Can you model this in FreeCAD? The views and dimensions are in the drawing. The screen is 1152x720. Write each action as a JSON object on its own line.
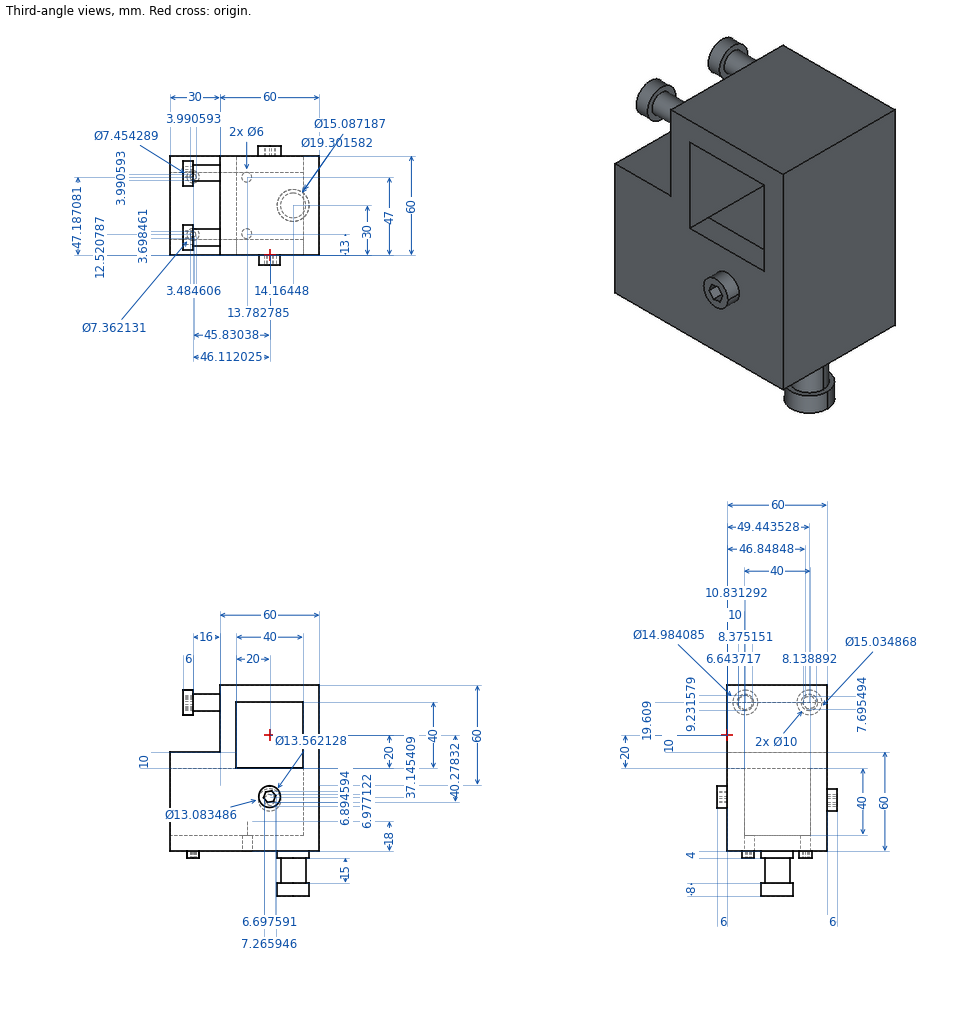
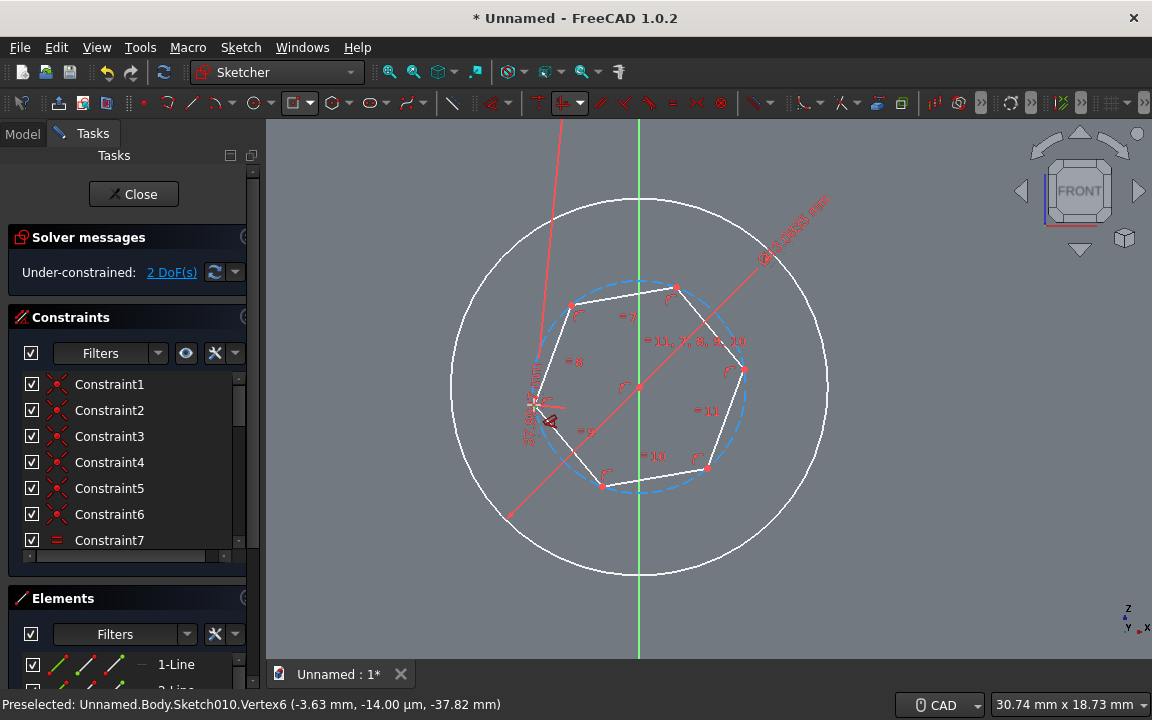
{"action": "left_click", "coordinate": [744, 369]}
{"action": "left_click", "coordinate": [591, 439]}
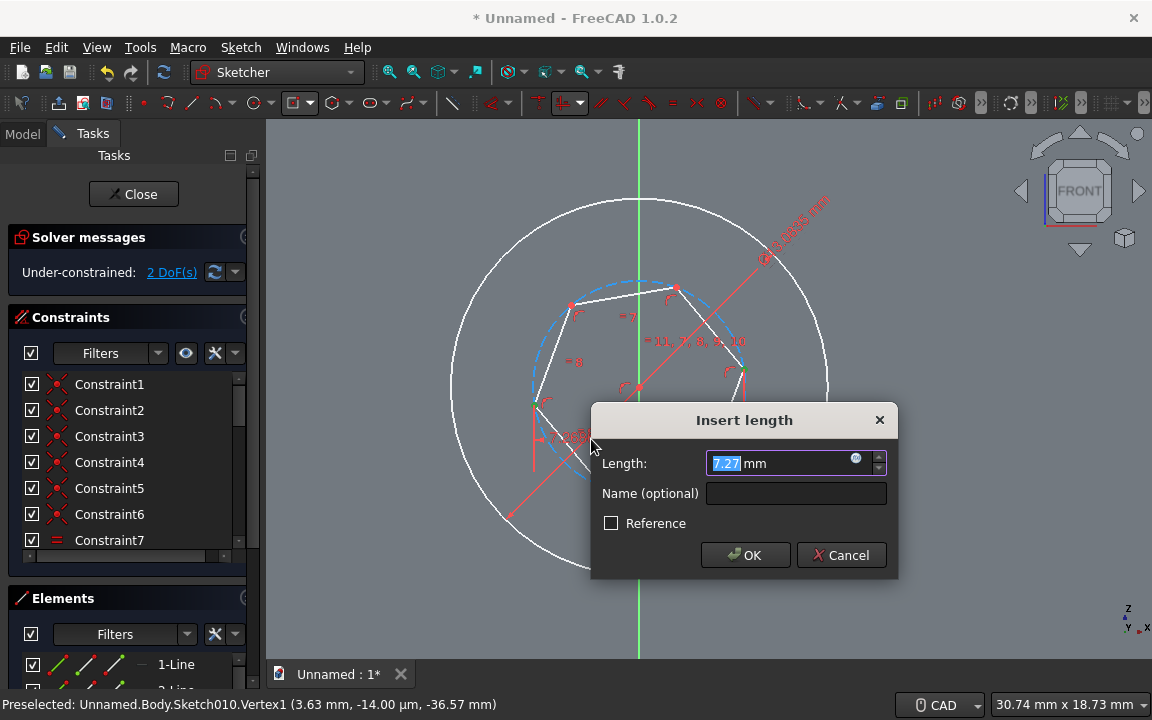
{"action": "type", "text": "7.265946"}
{"action": "key", "text": "Return"}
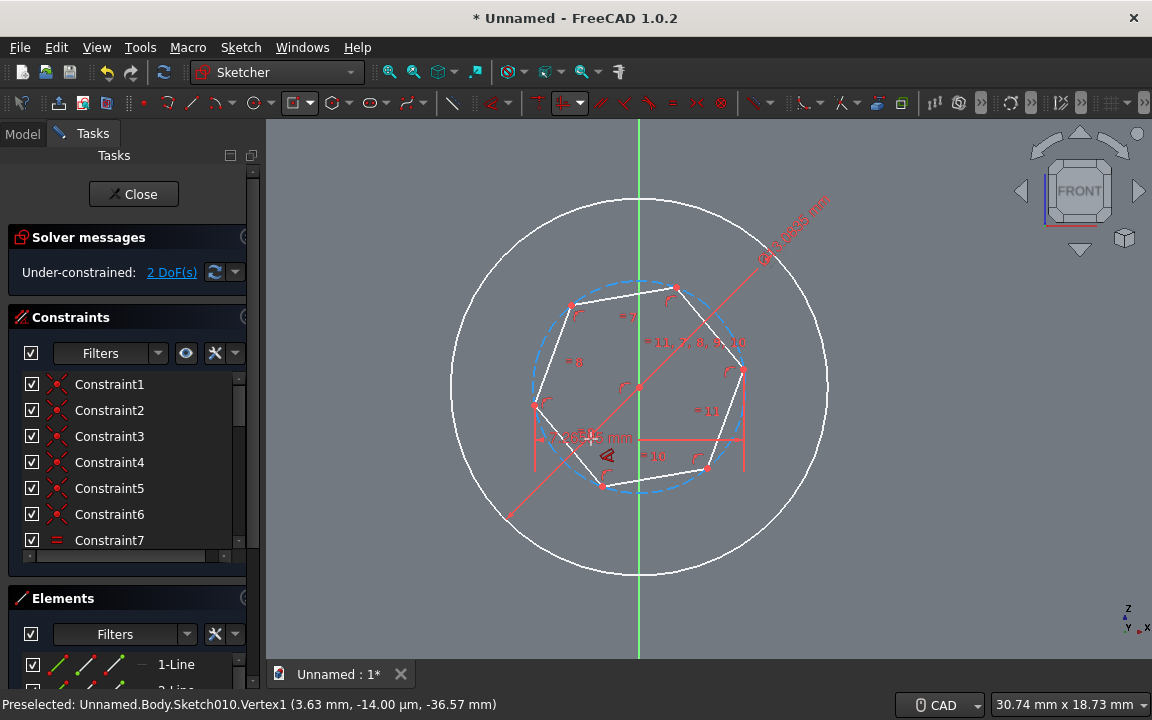
{"action": "left_click", "coordinate": [602, 487]}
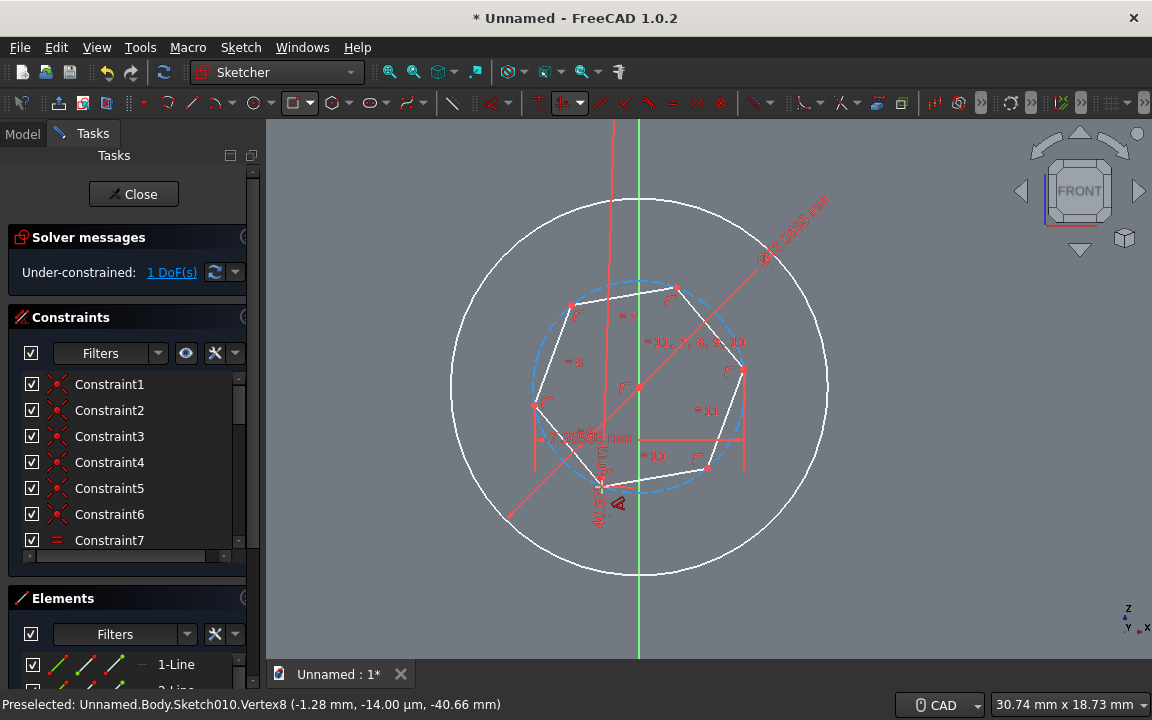
{"action": "left_click", "coordinate": [676, 287]}
{"action": "left_click", "coordinate": [710, 387]}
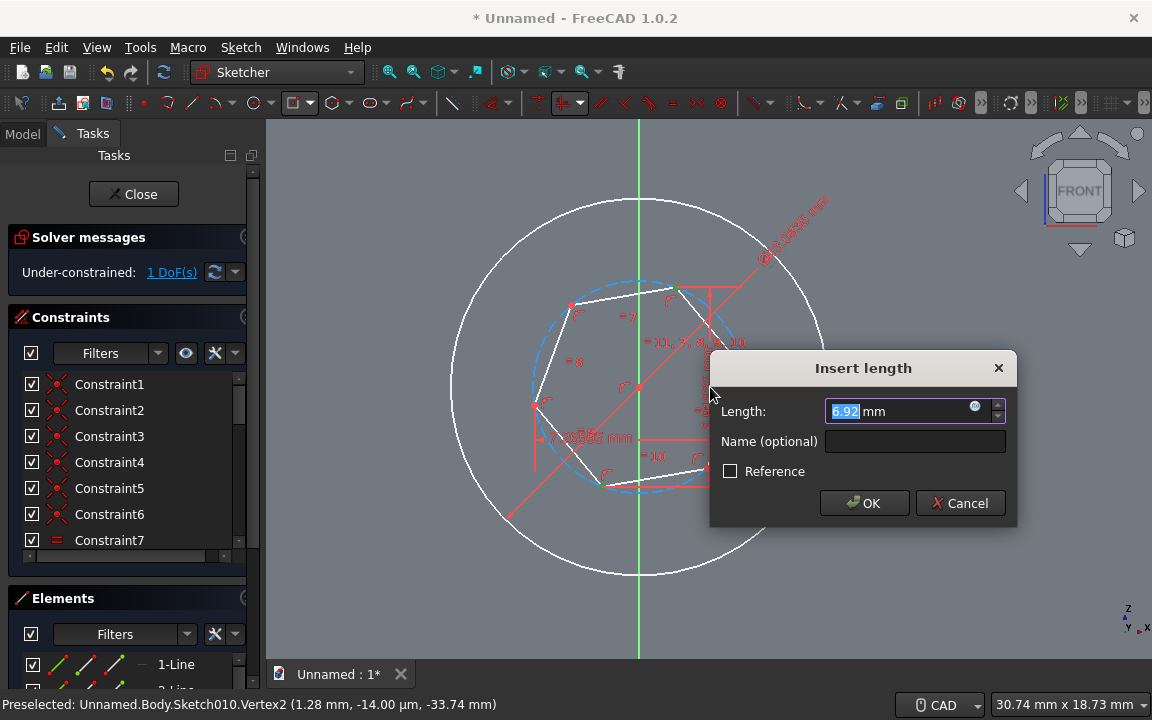
{"action": "type", "text": "6.894594"}
{"action": "key", "text": "Return"}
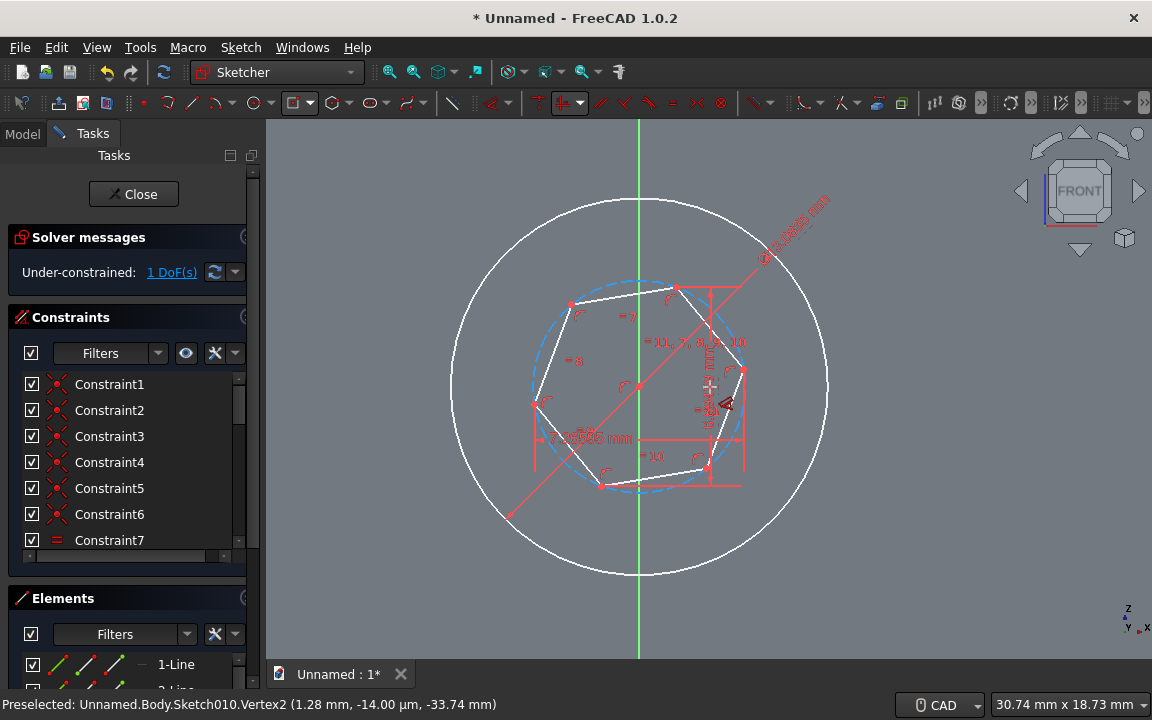
{"action": "left_click", "coordinate": [639, 387]}
{"action": "left_click", "coordinate": [673, 267]}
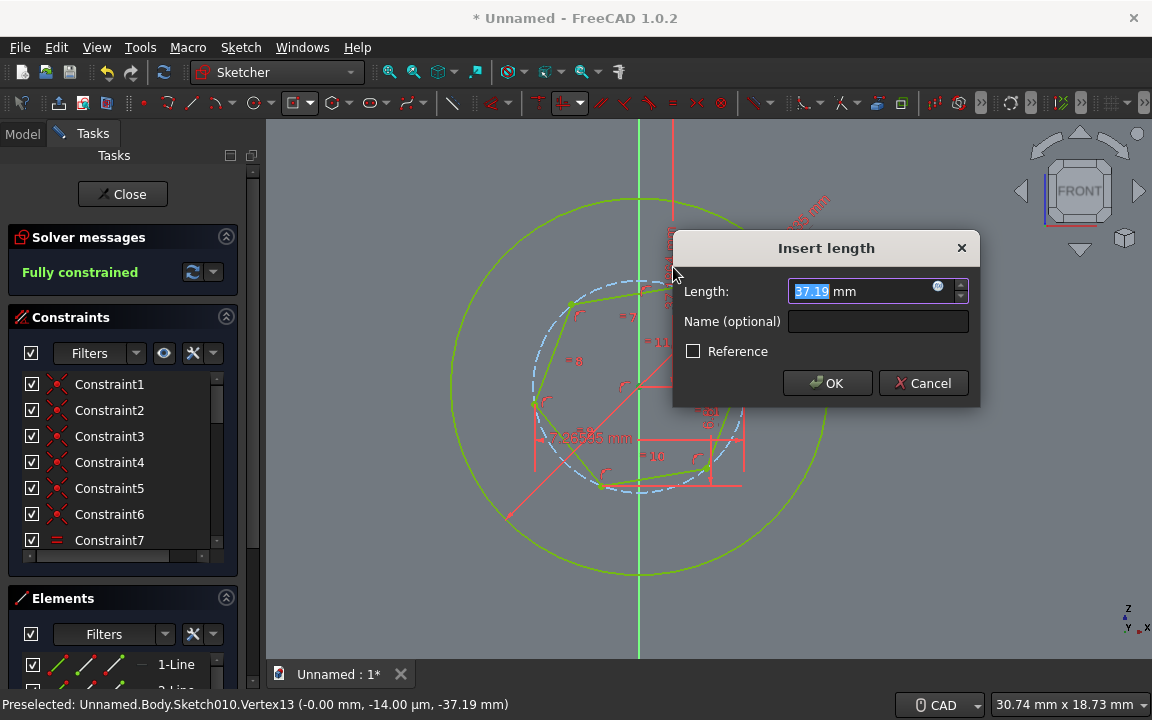
{"action": "type", "text": "37.145409"}
{"action": "key", "text": "Return"}
{"action": "key", "text": "Escape"}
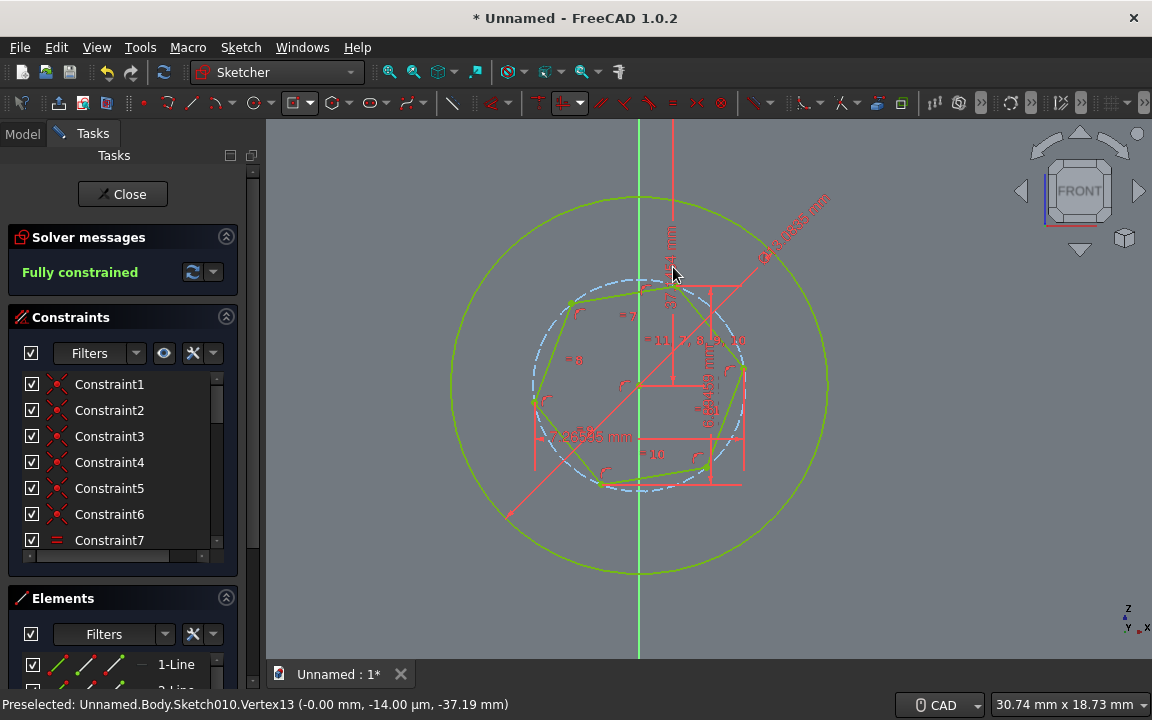
{"action": "left_click", "coordinate": [123, 194]}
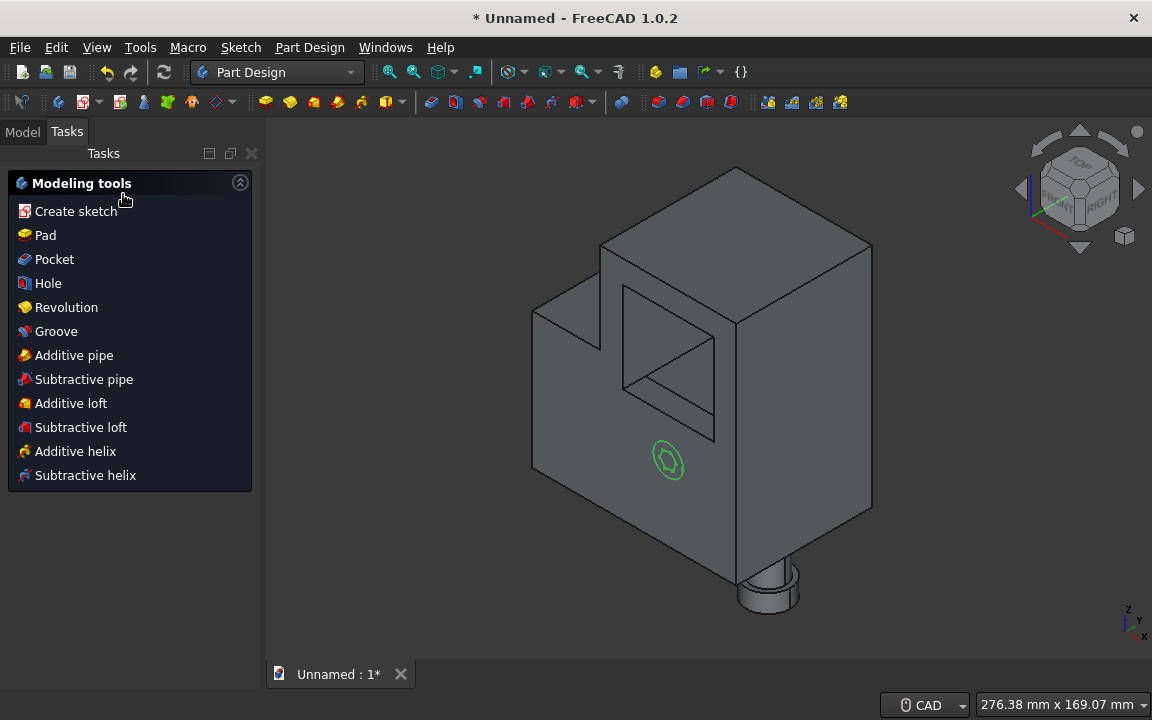
{"action": "left_click", "coordinate": [266, 102]}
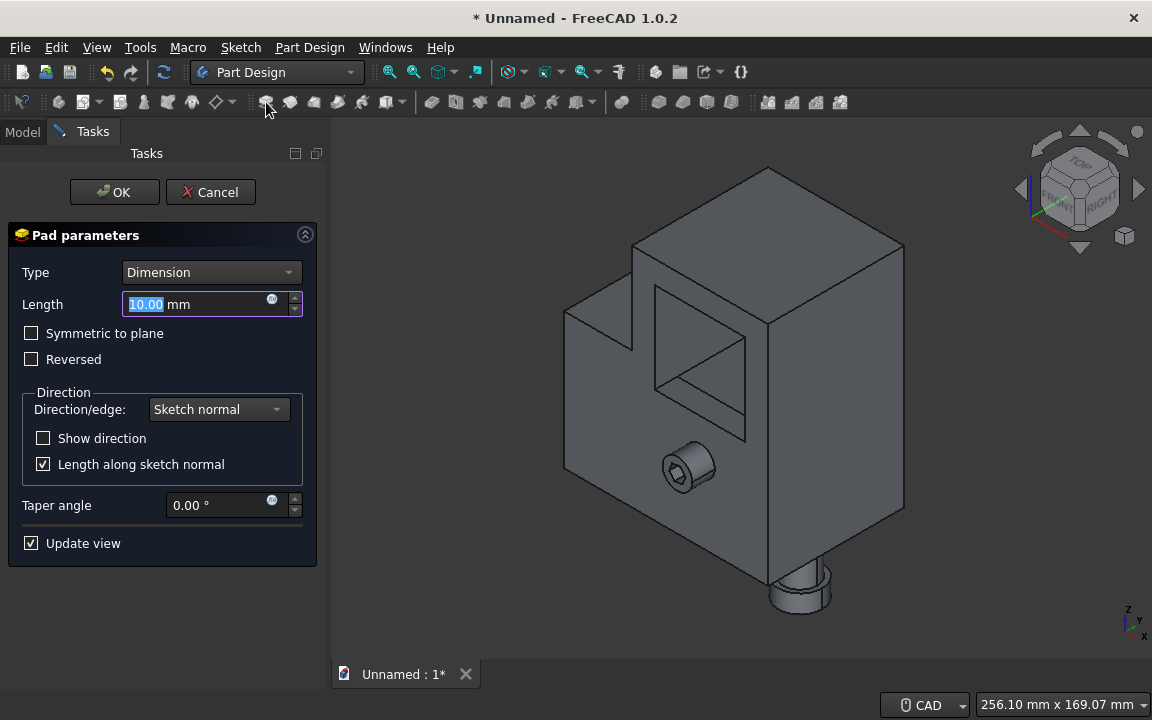
{"action": "type", "text": "6"}
{"action": "key", "text": "Tab"}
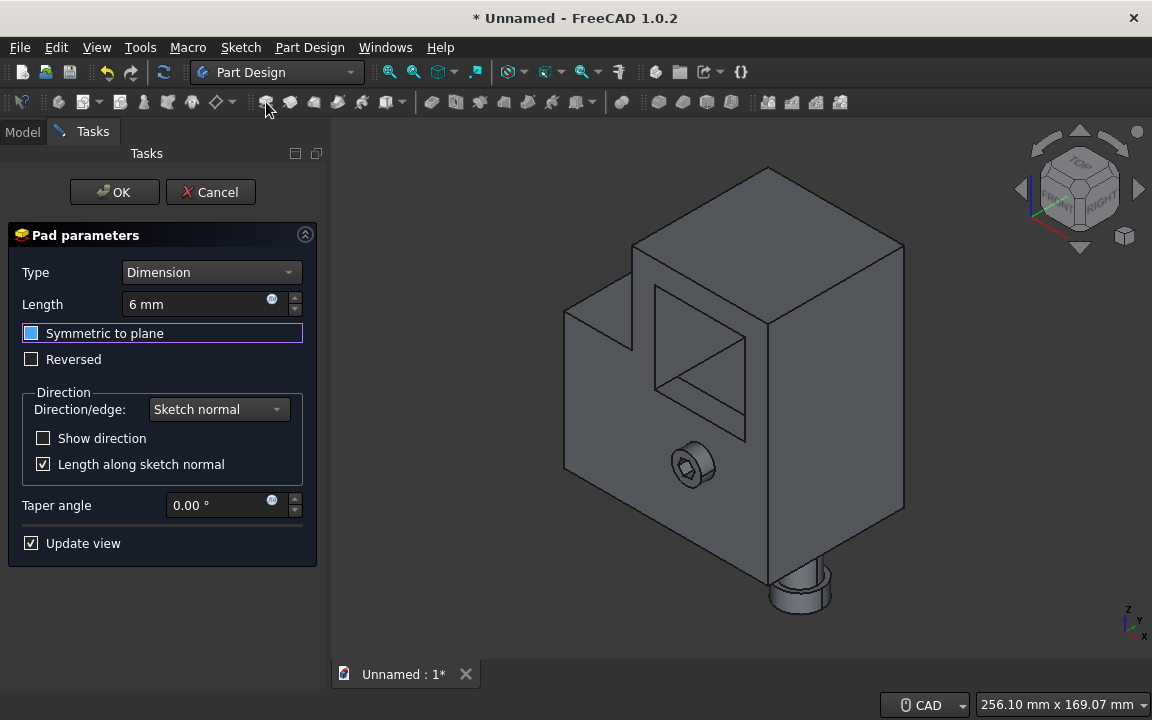
{"action": "left_click", "coordinate": [115, 192]}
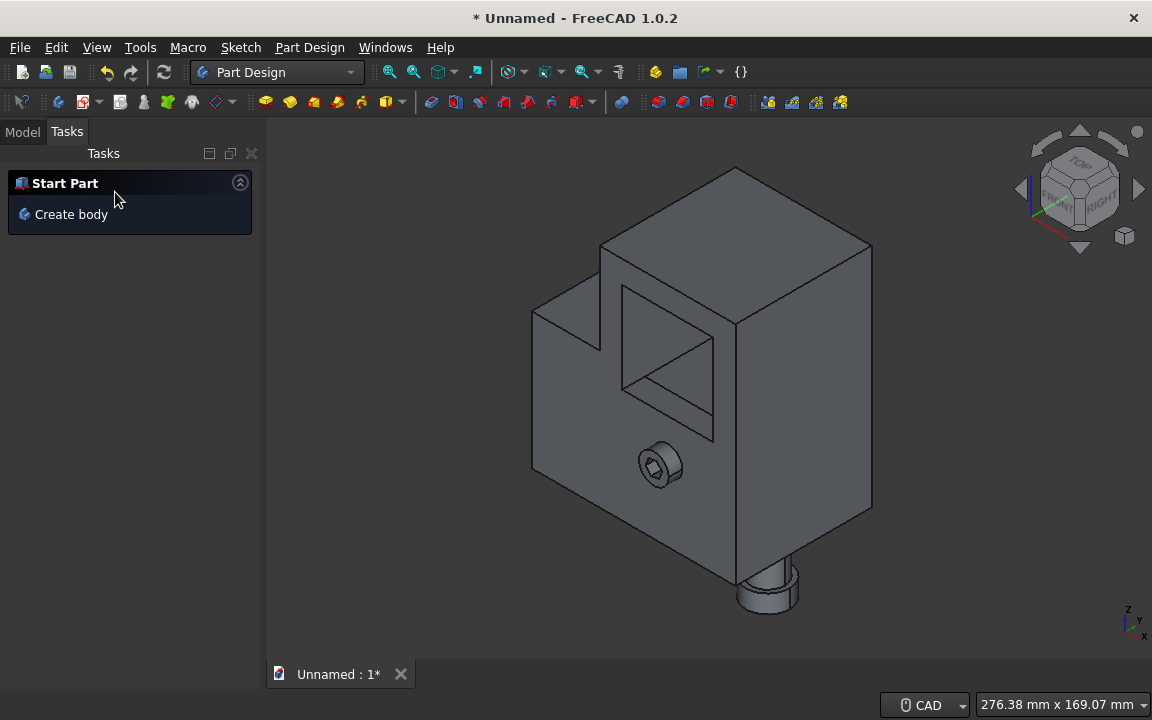
{"action": "left_click", "coordinate": [390, 72]}